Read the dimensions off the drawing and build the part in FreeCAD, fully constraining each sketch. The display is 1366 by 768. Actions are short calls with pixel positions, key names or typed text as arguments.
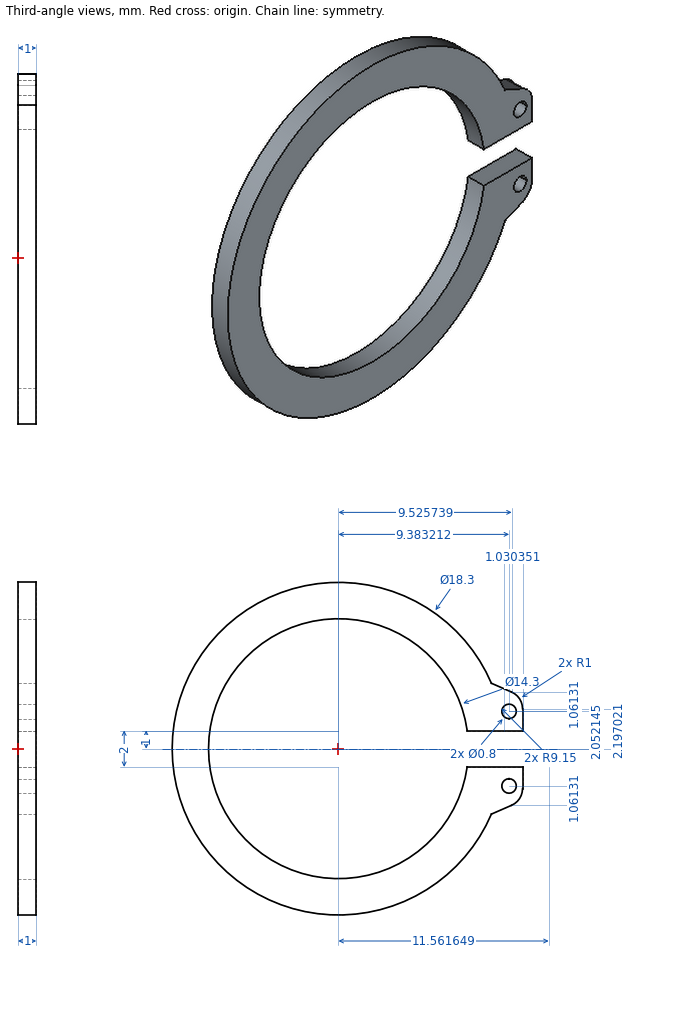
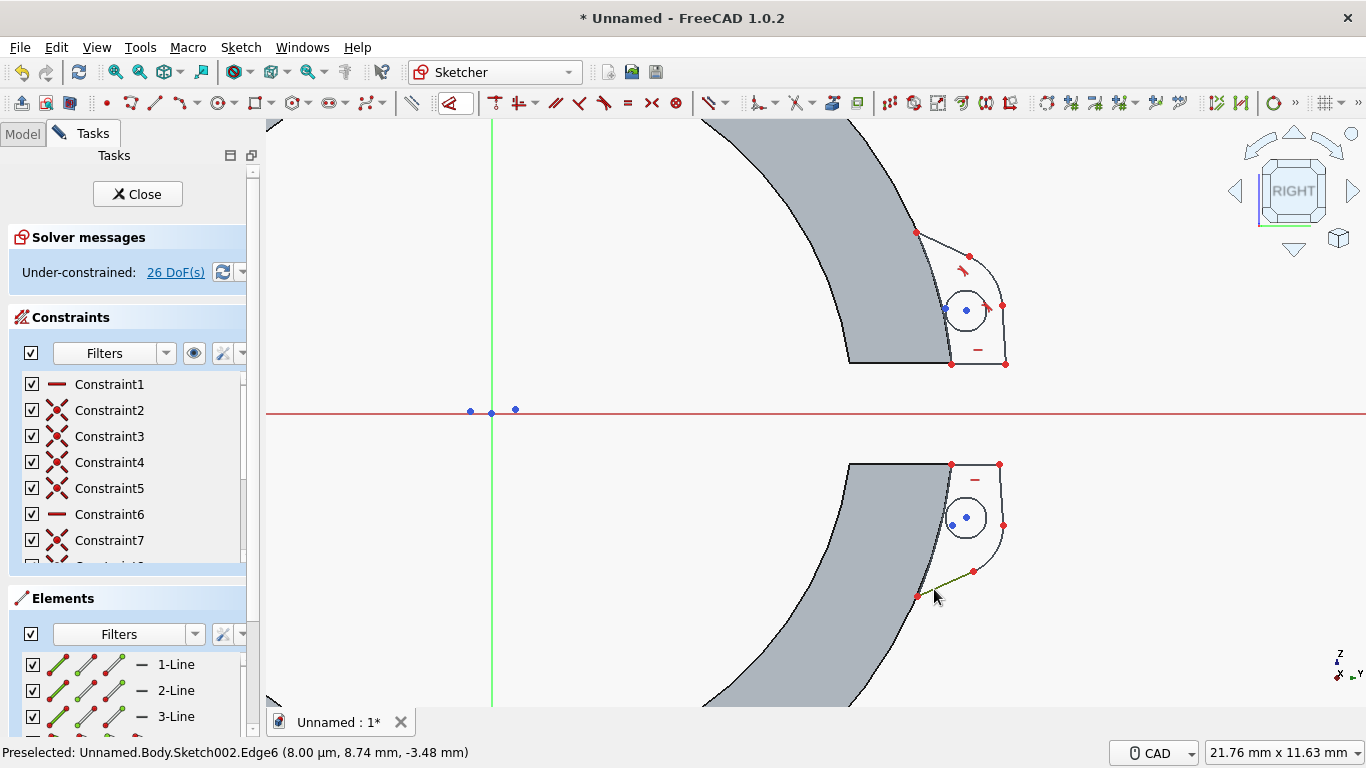
click(988, 562)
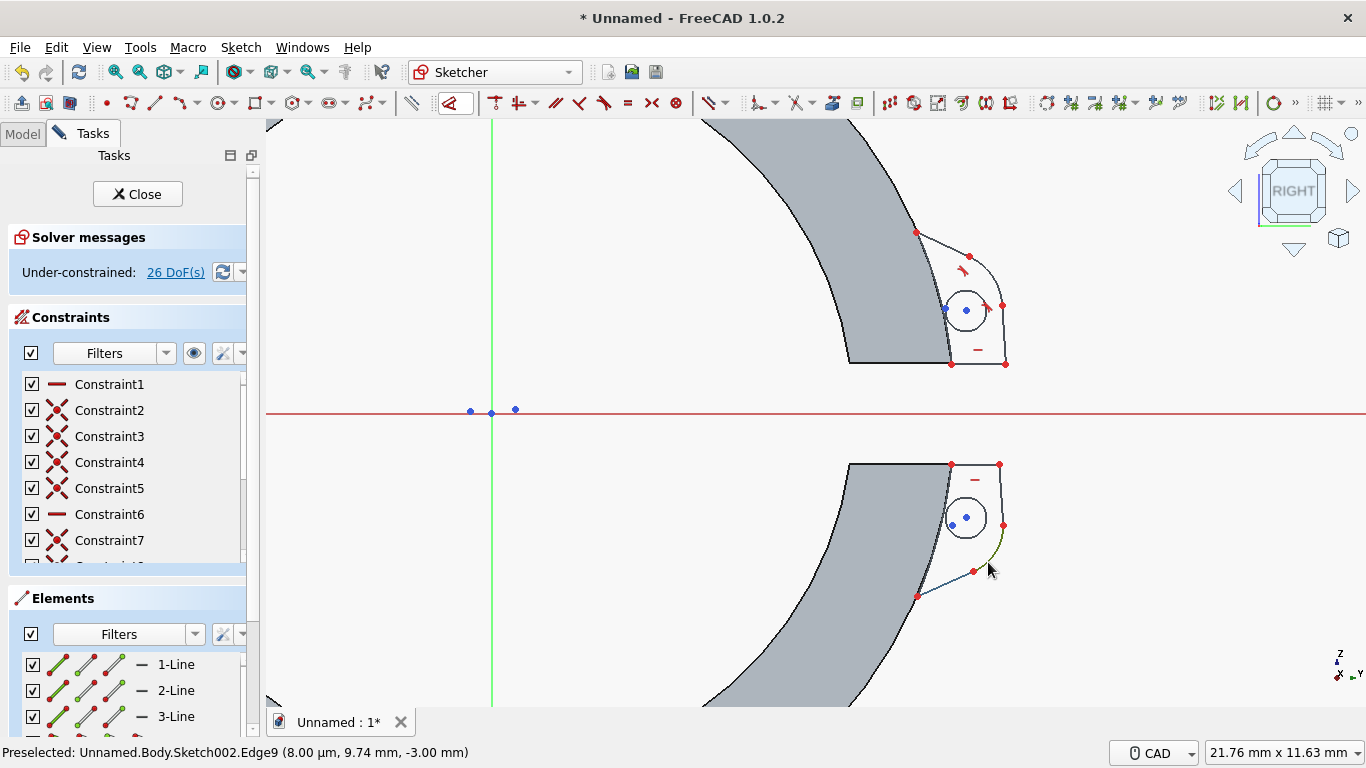
click(604, 104)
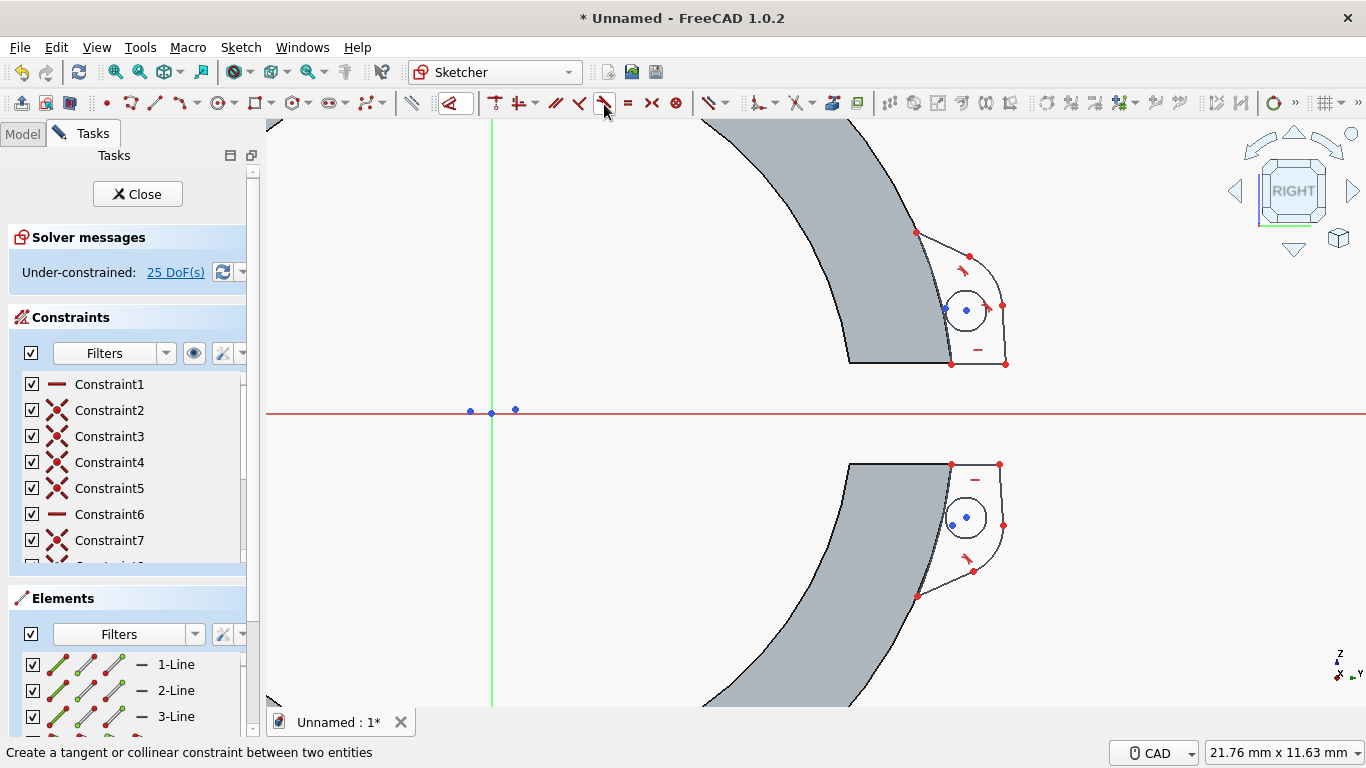
click(1002, 508)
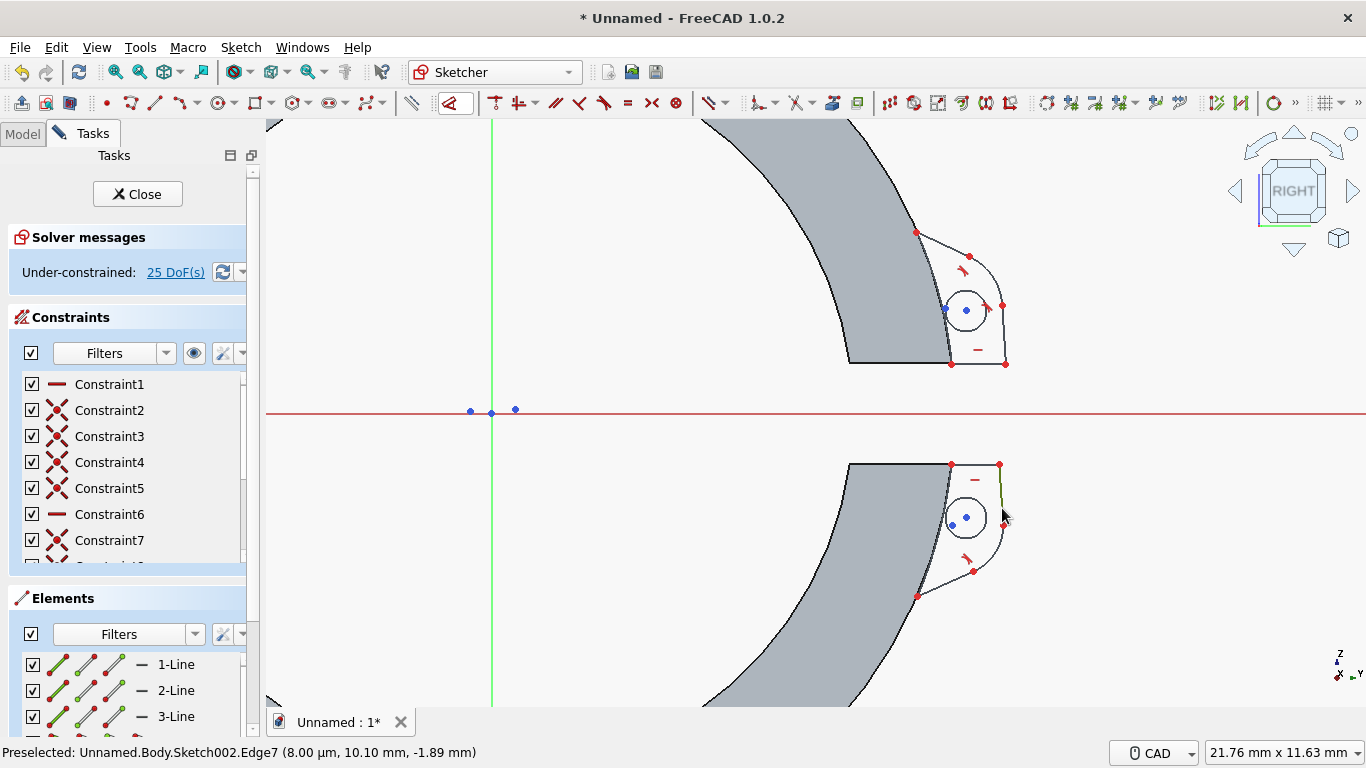
click(988, 562)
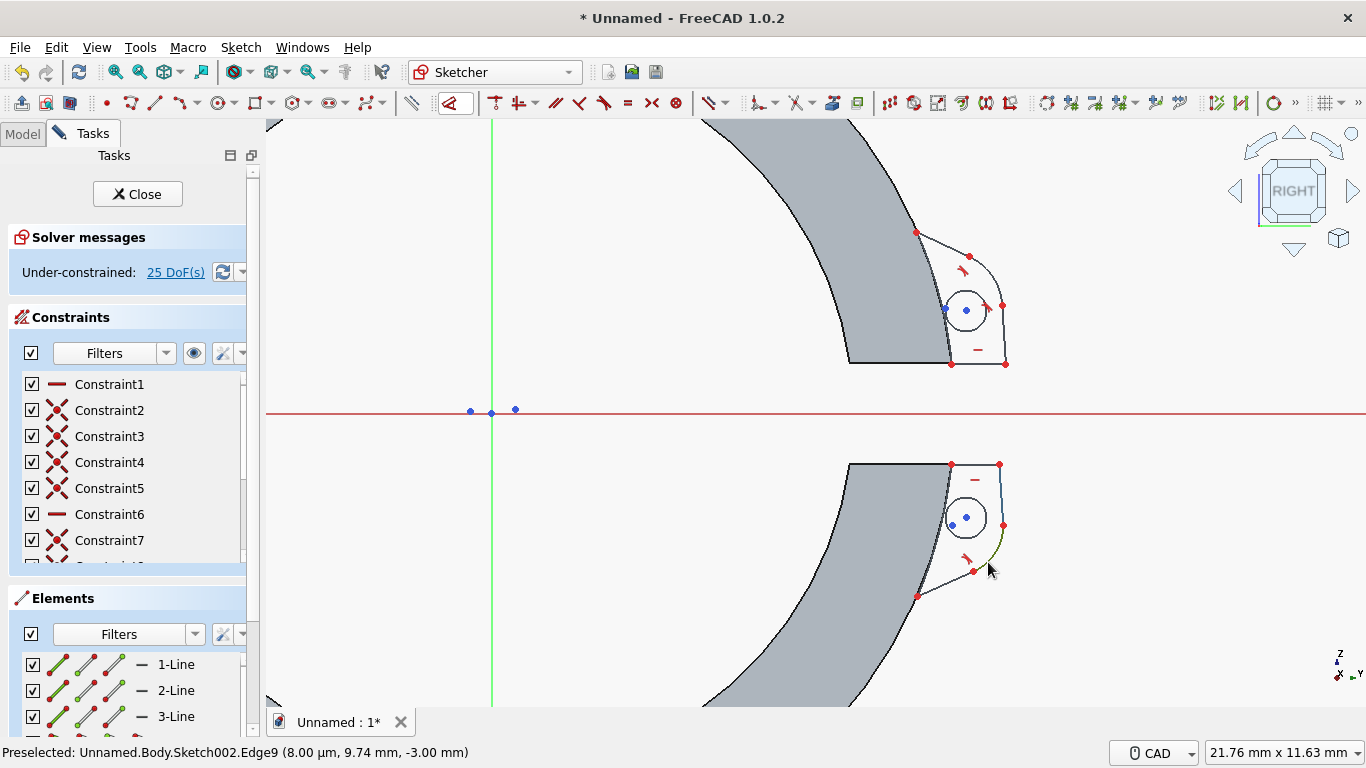
click(604, 104)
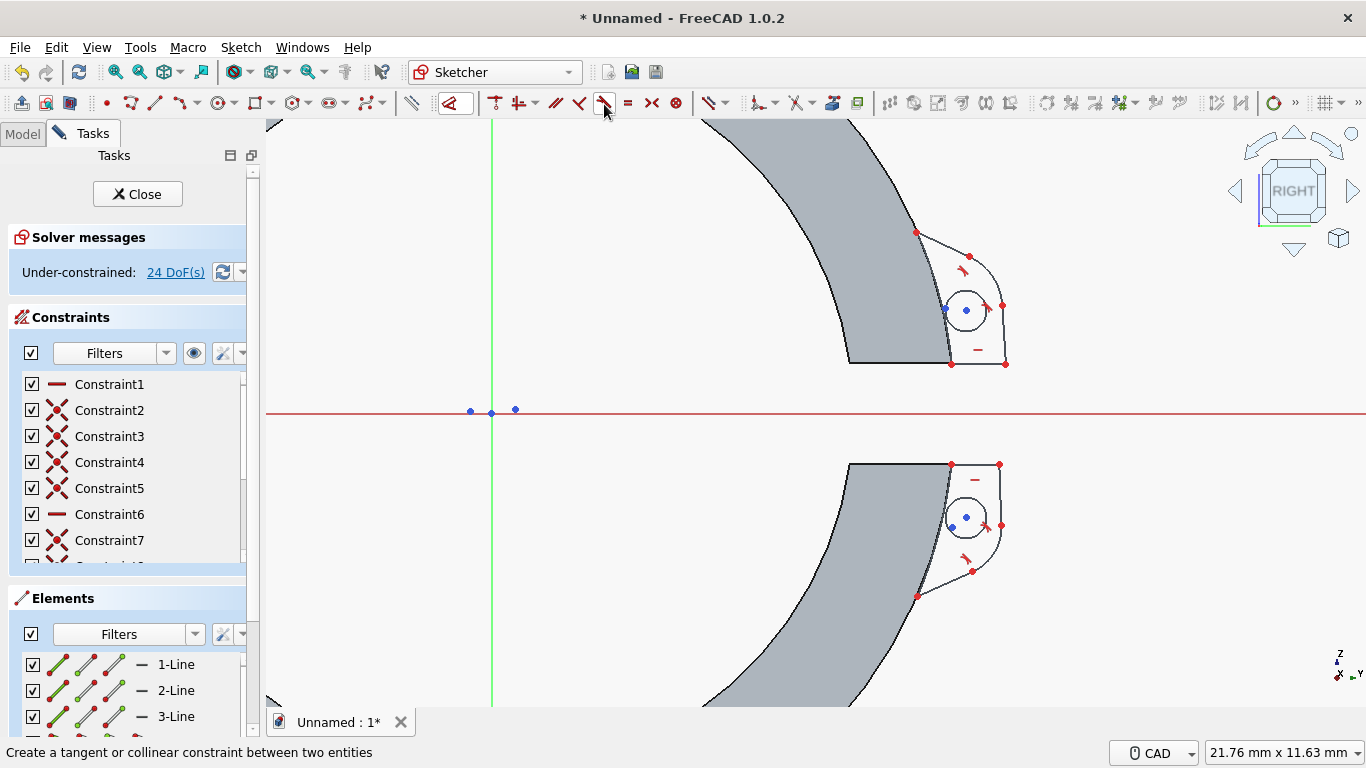
click(932, 270)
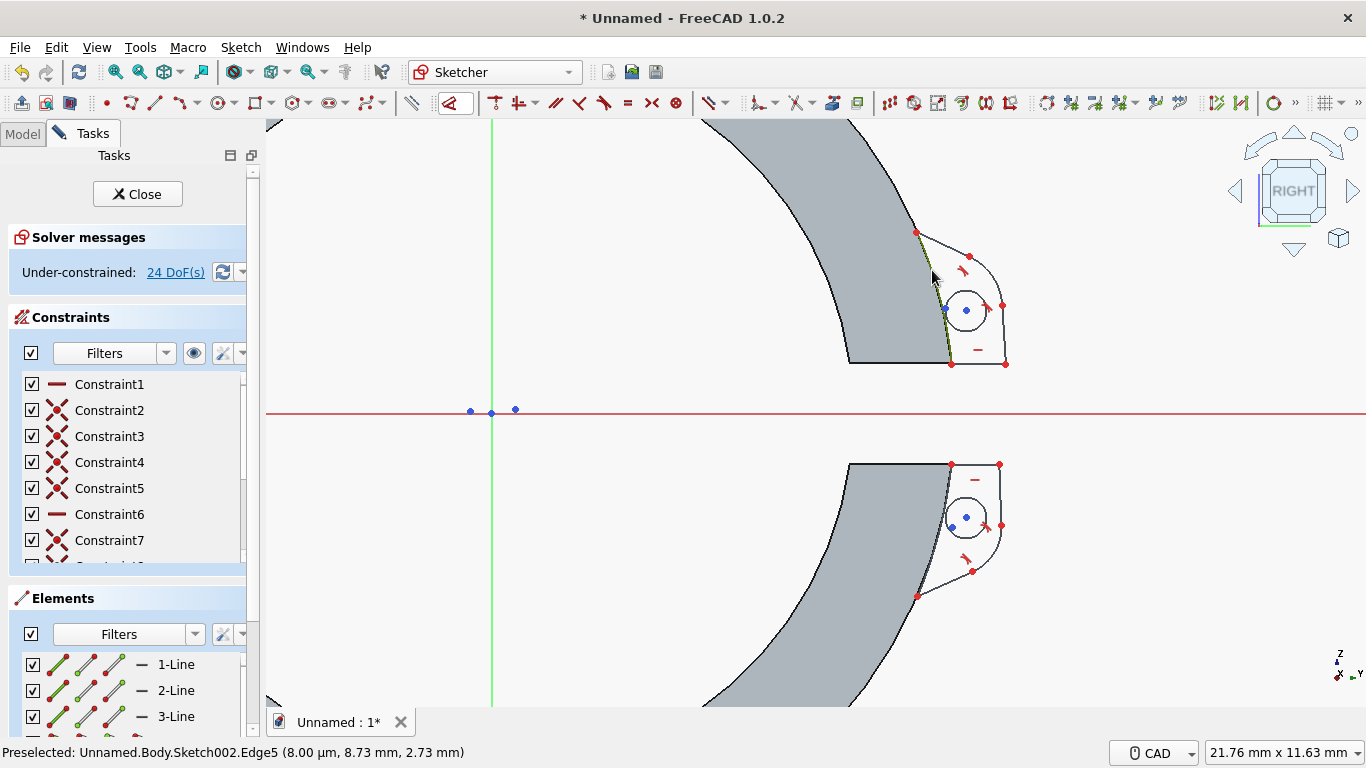
click(932, 558)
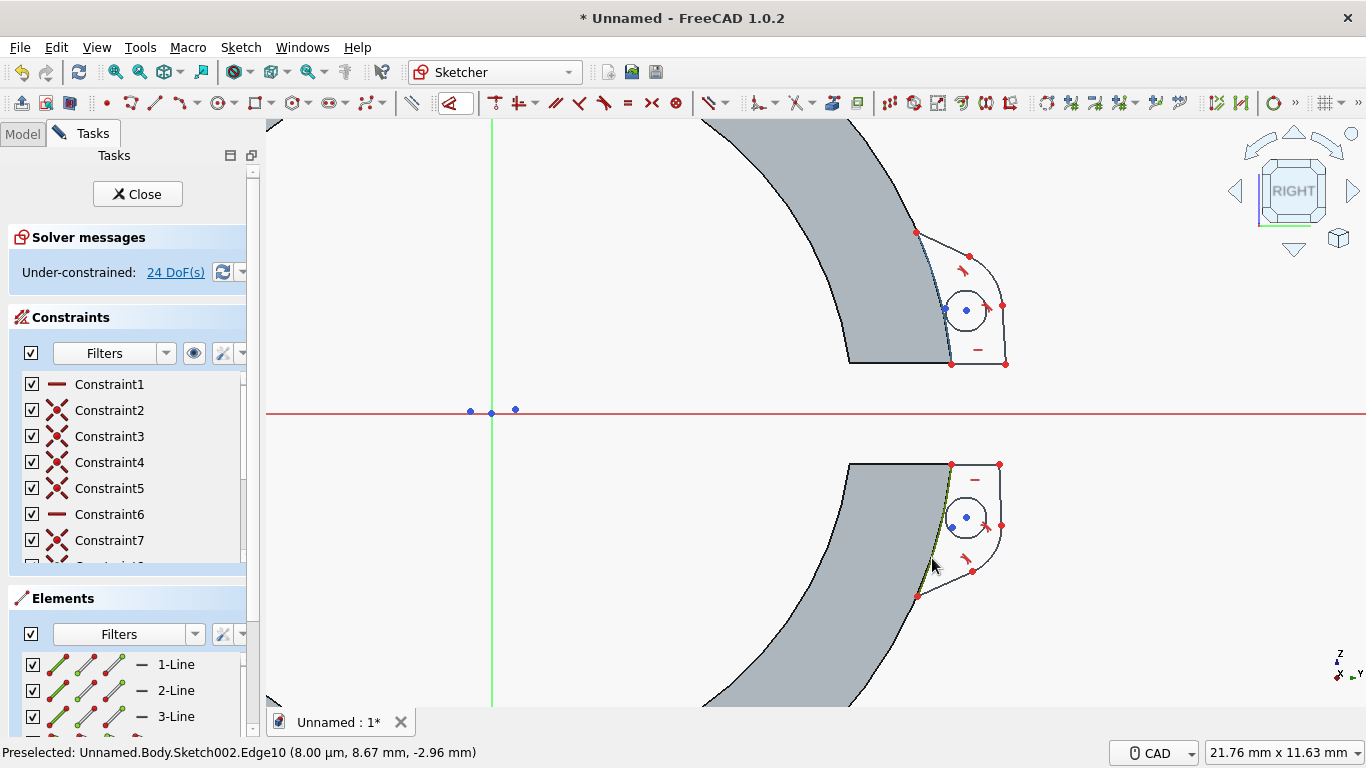
click(496, 104)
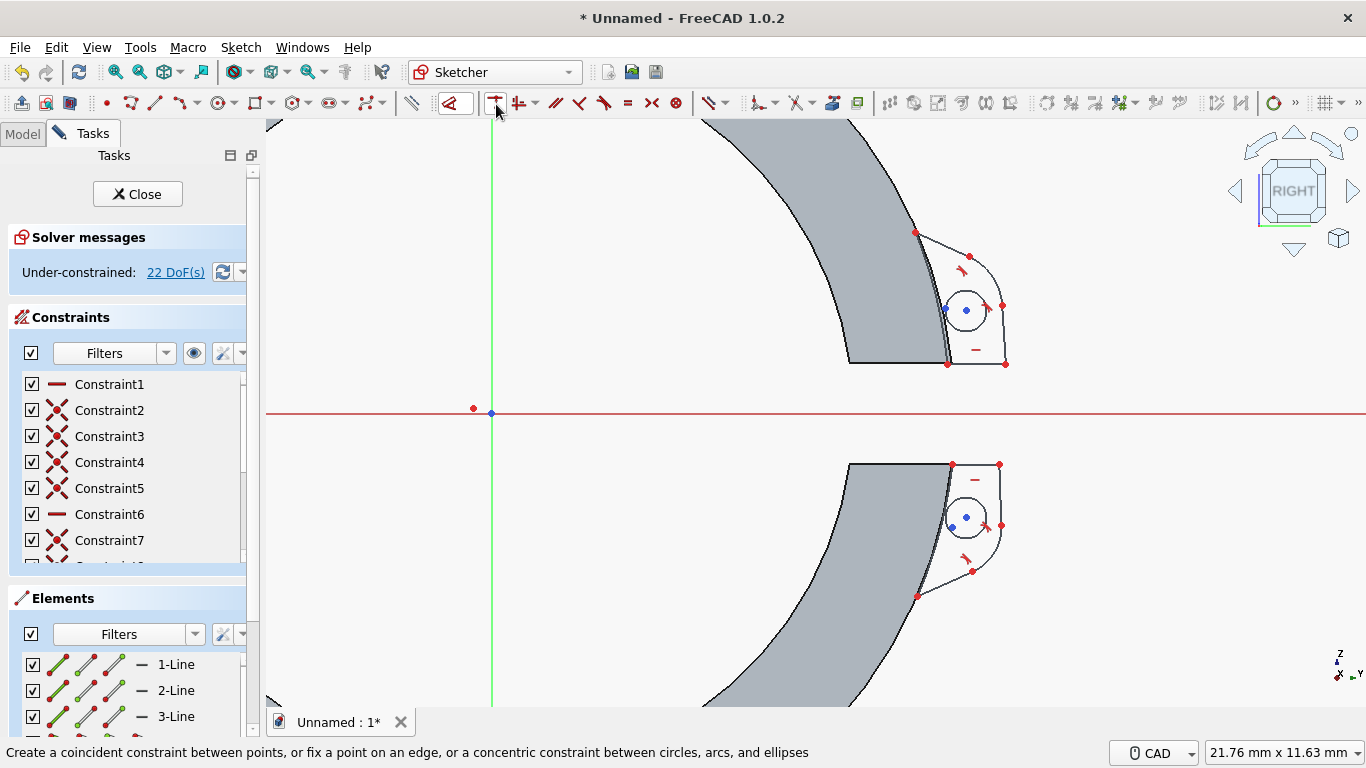
scroll(483, 411, up, 4)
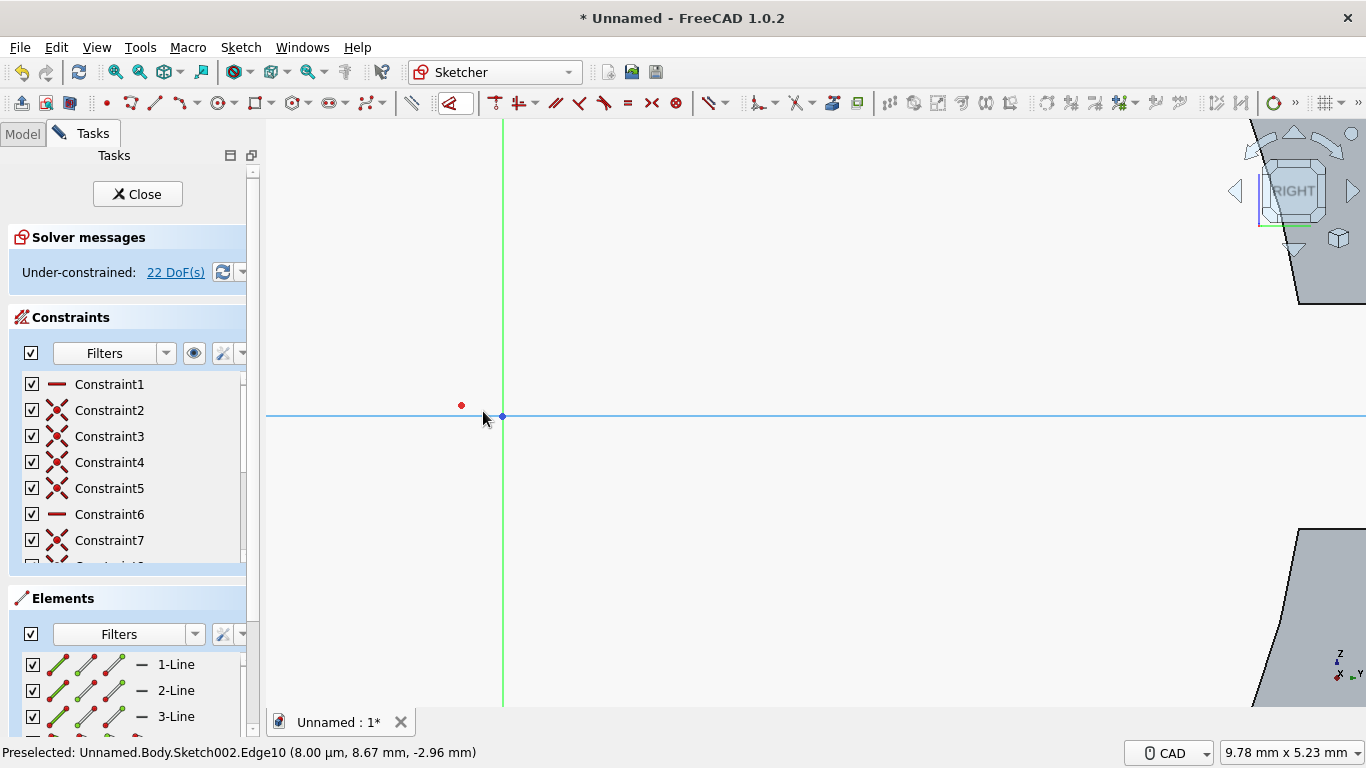
drag(452, 395, 513, 426)